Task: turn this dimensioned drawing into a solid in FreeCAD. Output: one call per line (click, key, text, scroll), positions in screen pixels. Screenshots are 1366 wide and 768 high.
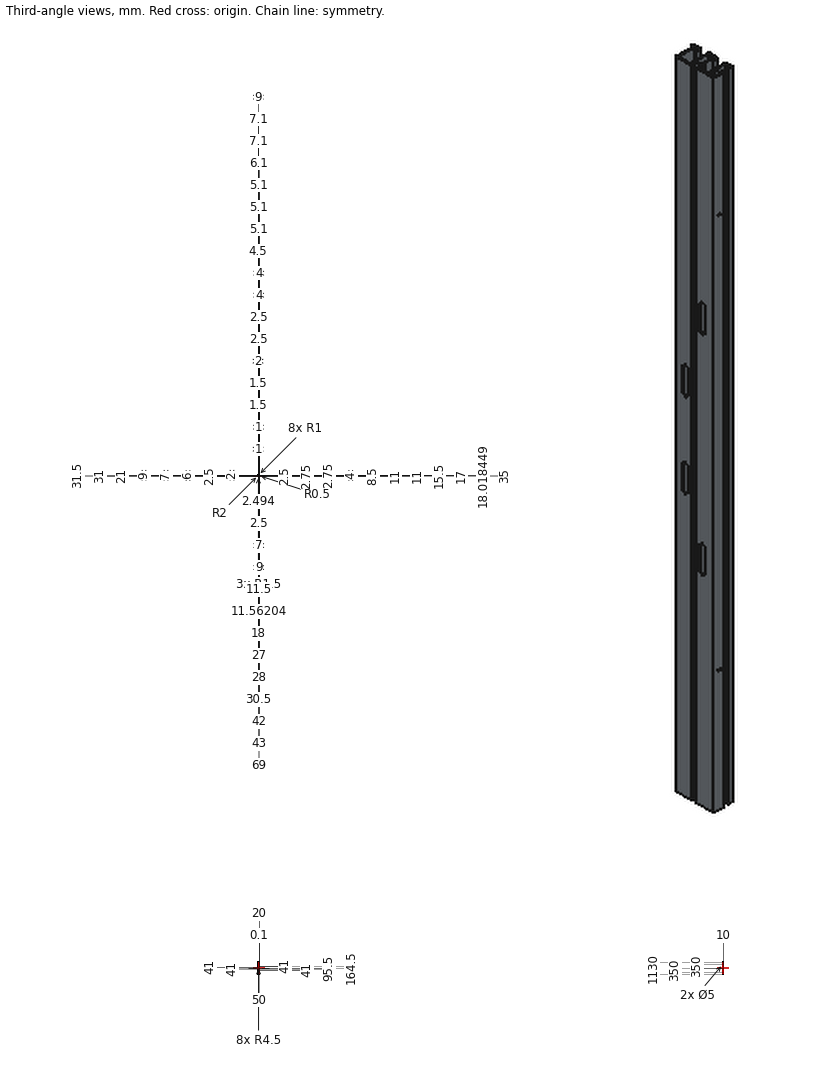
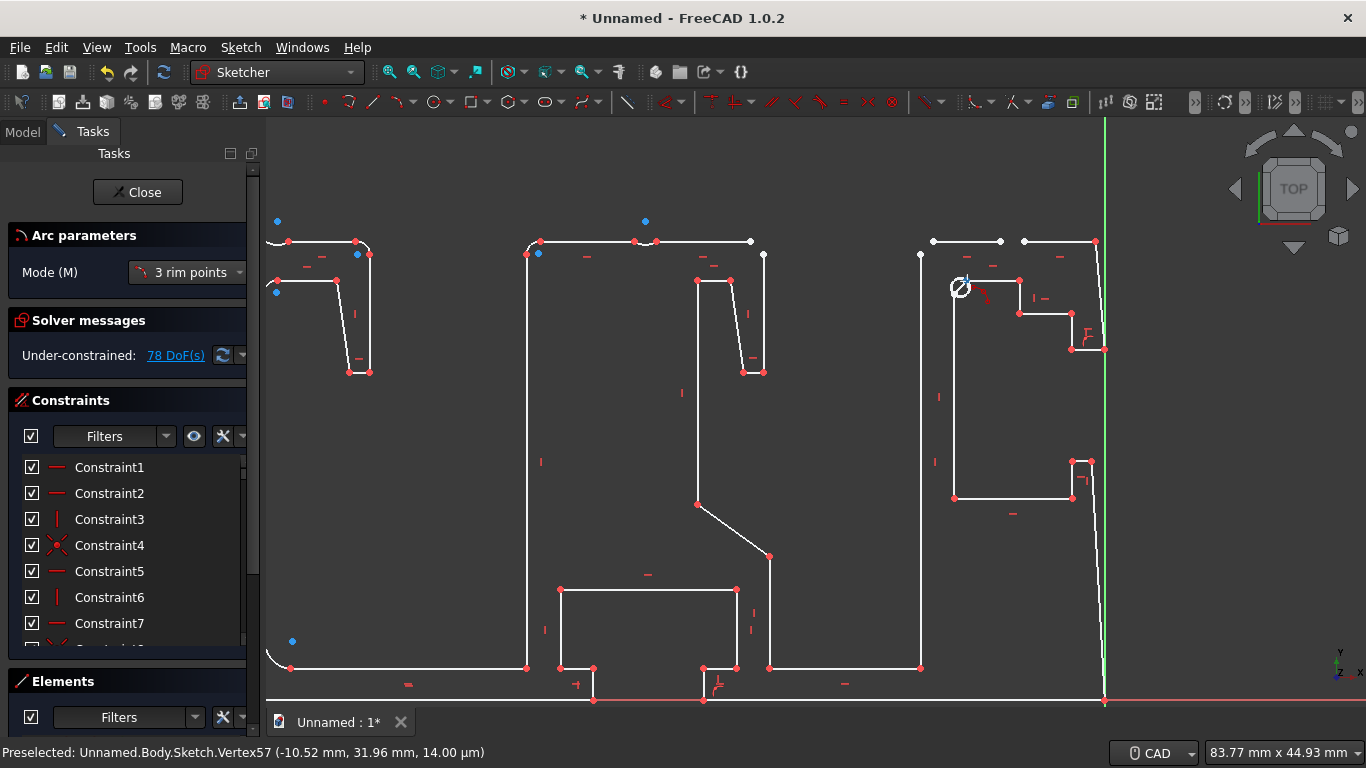
scroll(958, 284, up, 8)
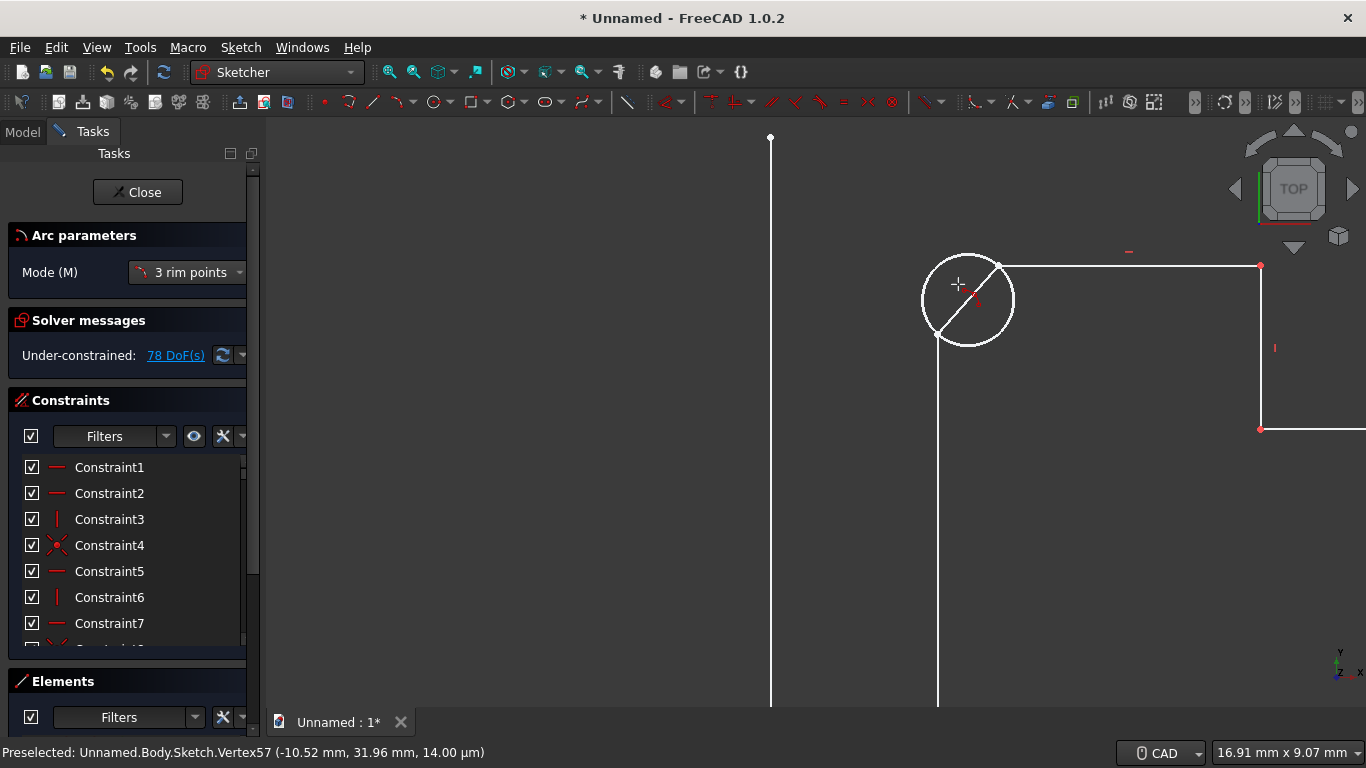
click(954, 282)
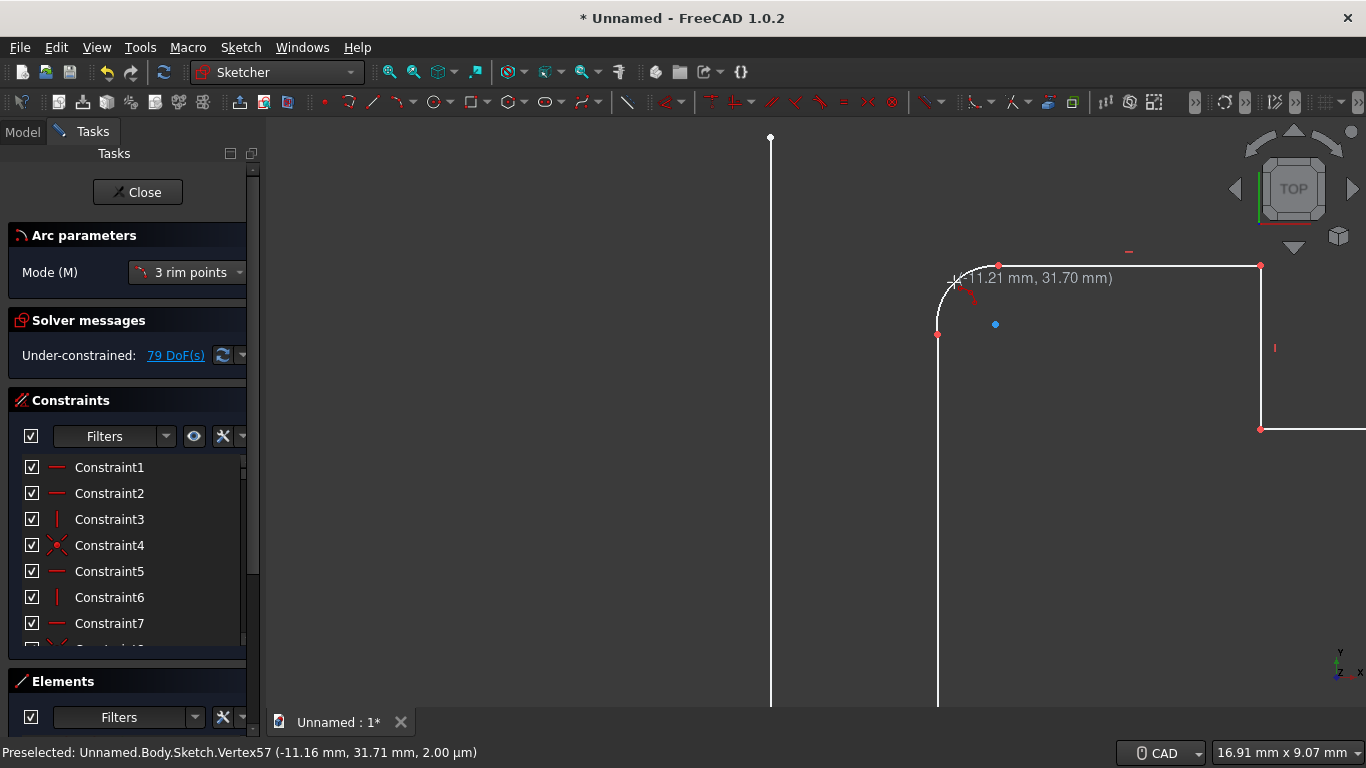
scroll(957, 288, down, 10)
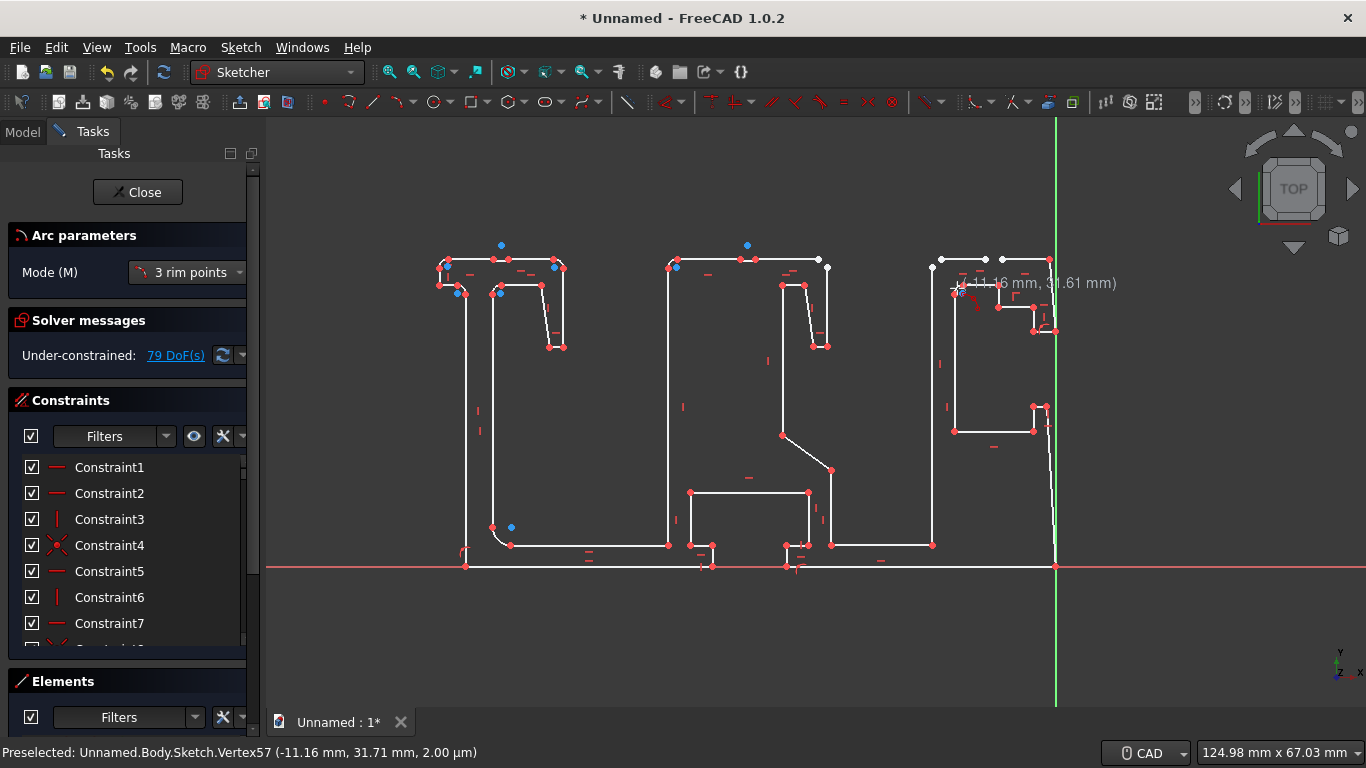
click(1002, 259)
click(986, 259)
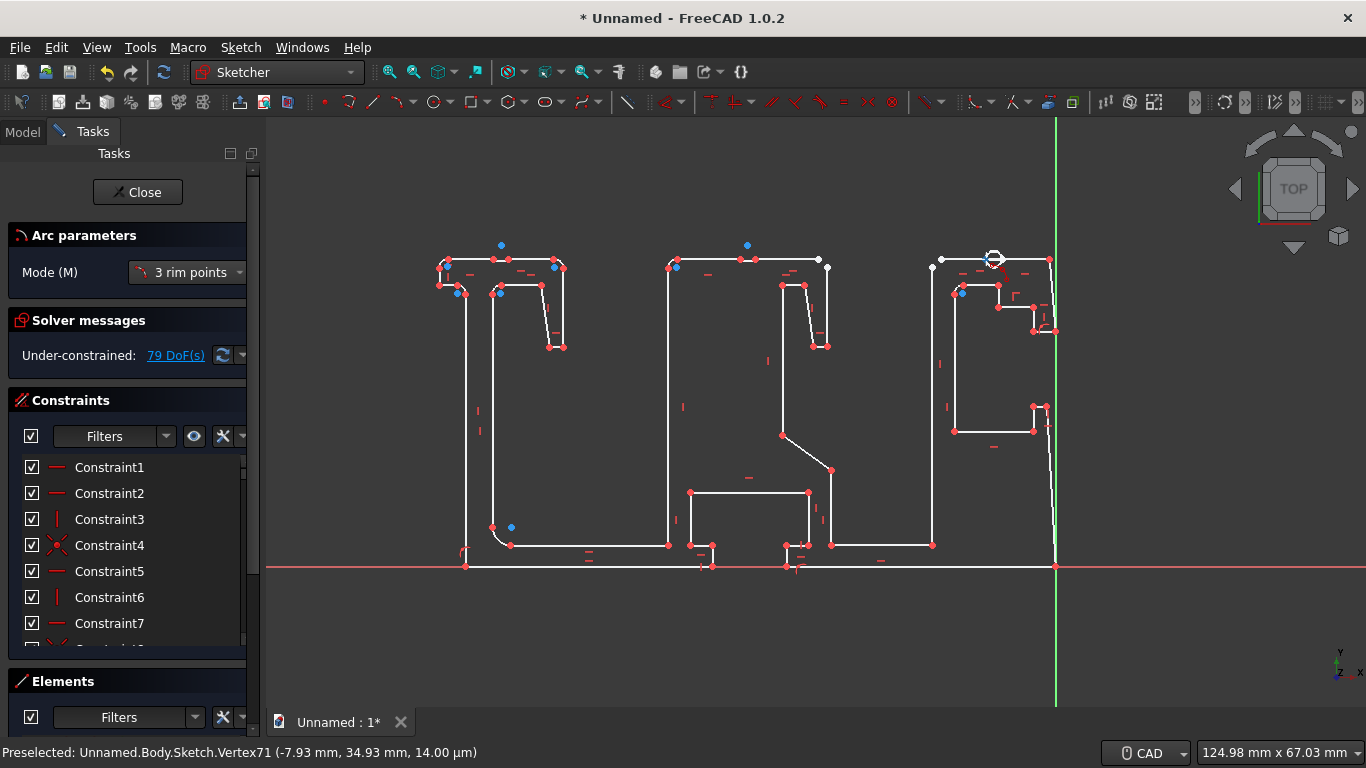
scroll(994, 261, up, 9)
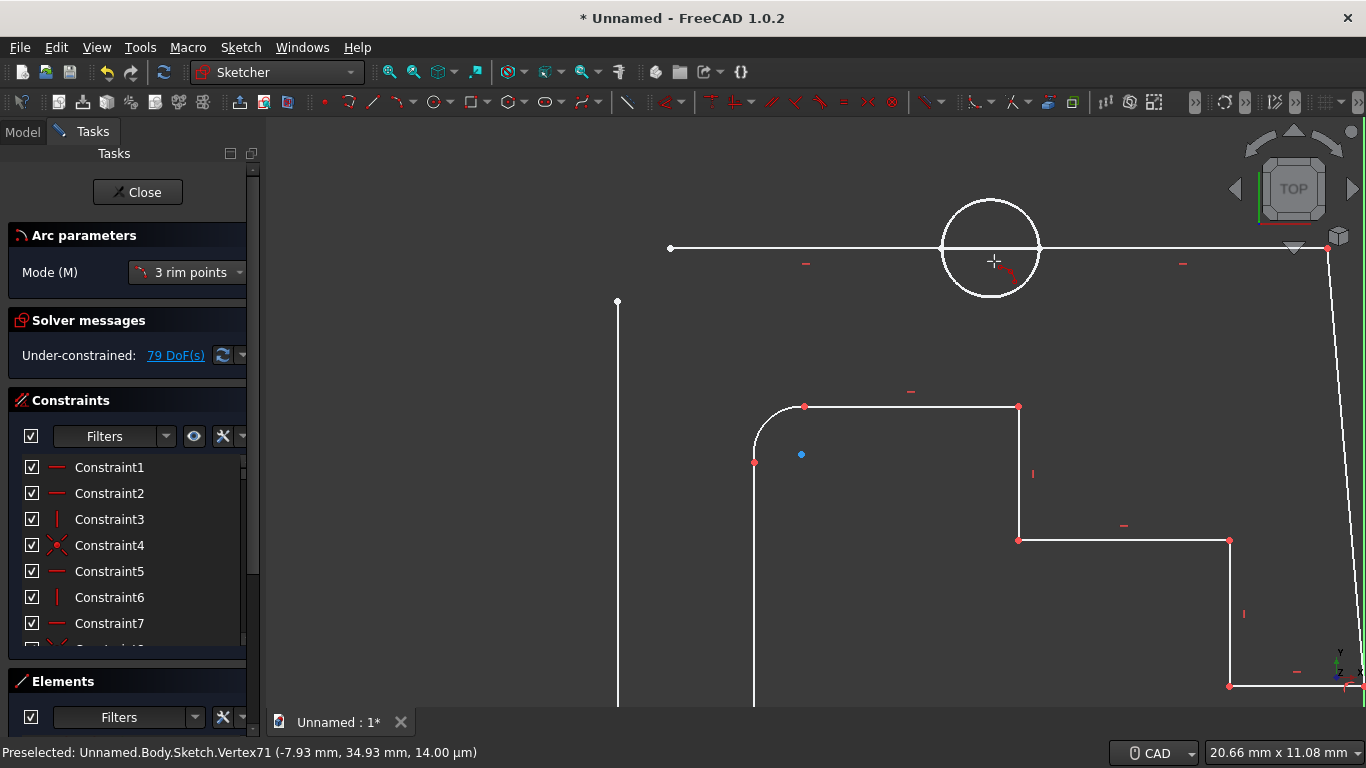
click(992, 261)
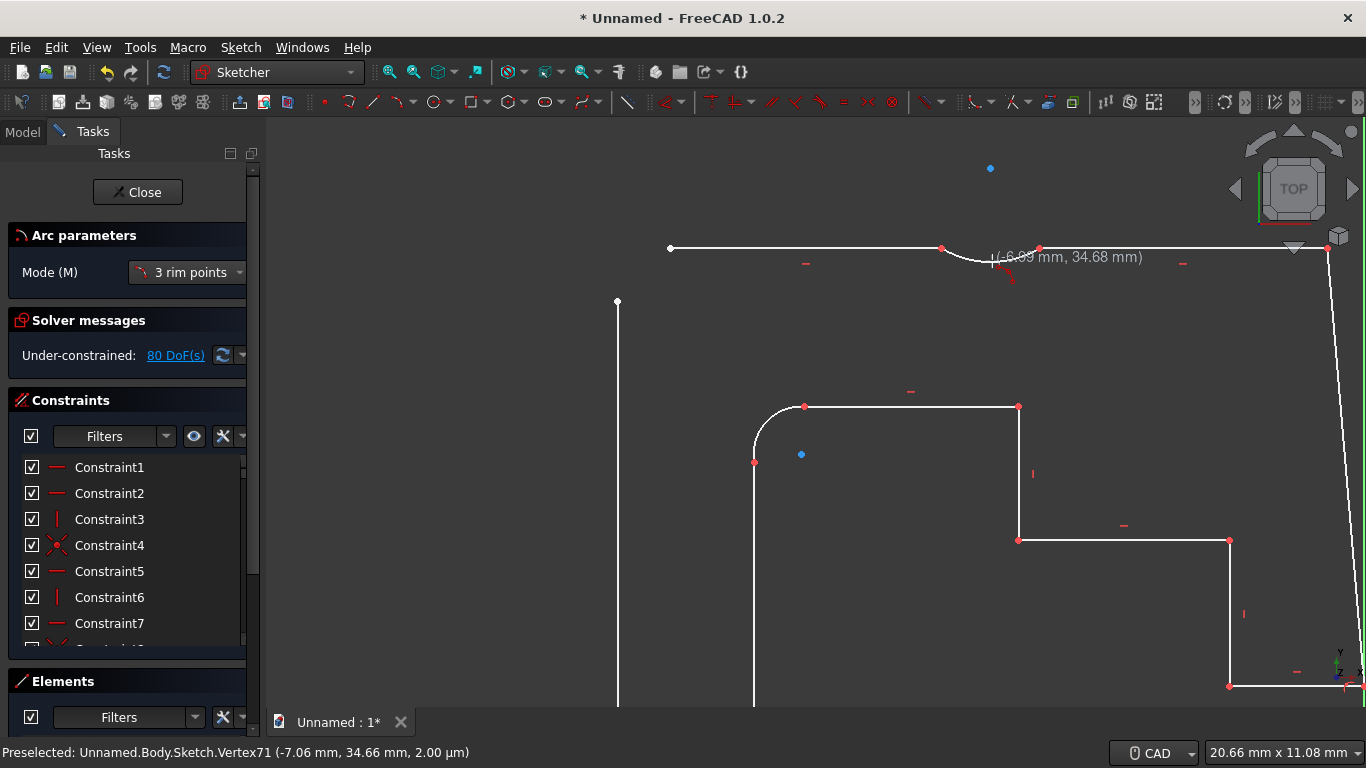
scroll(994, 261, down, 9)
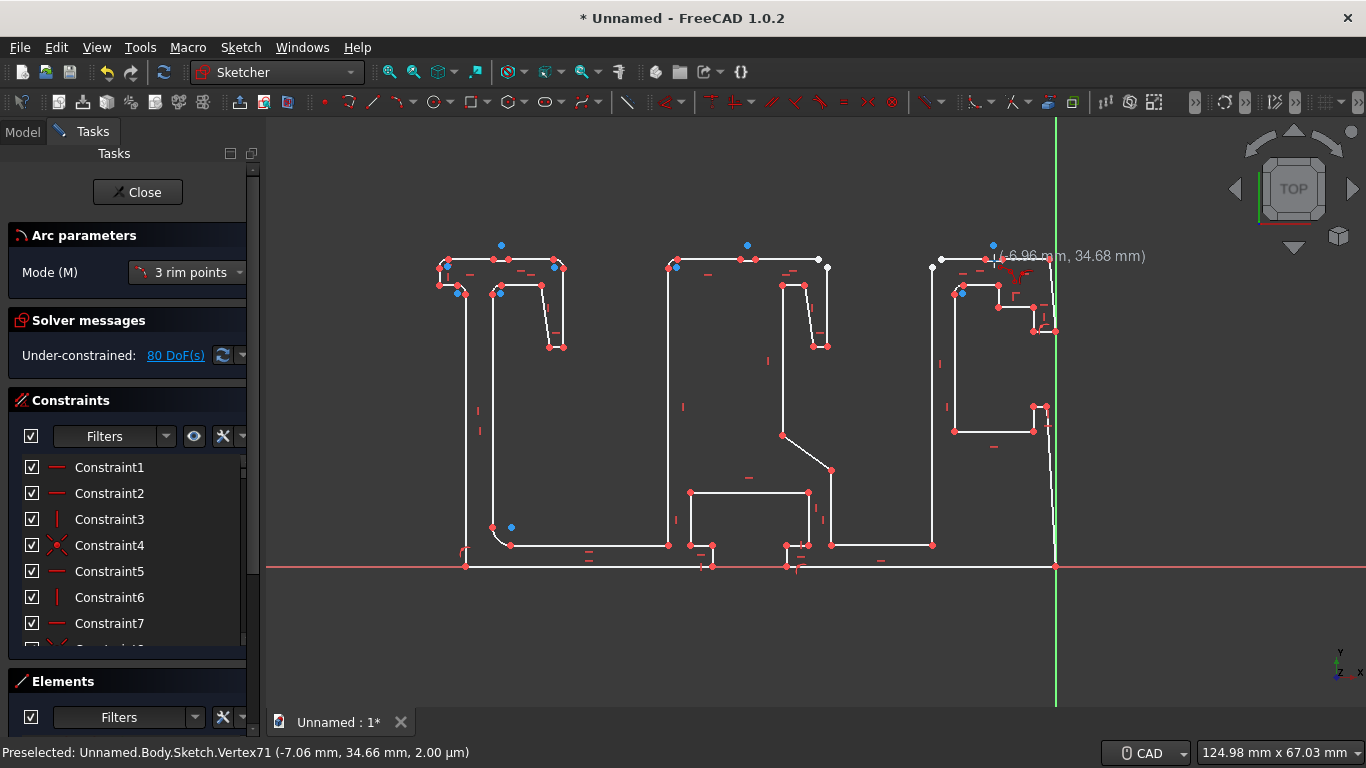
scroll(941, 259, up, 2)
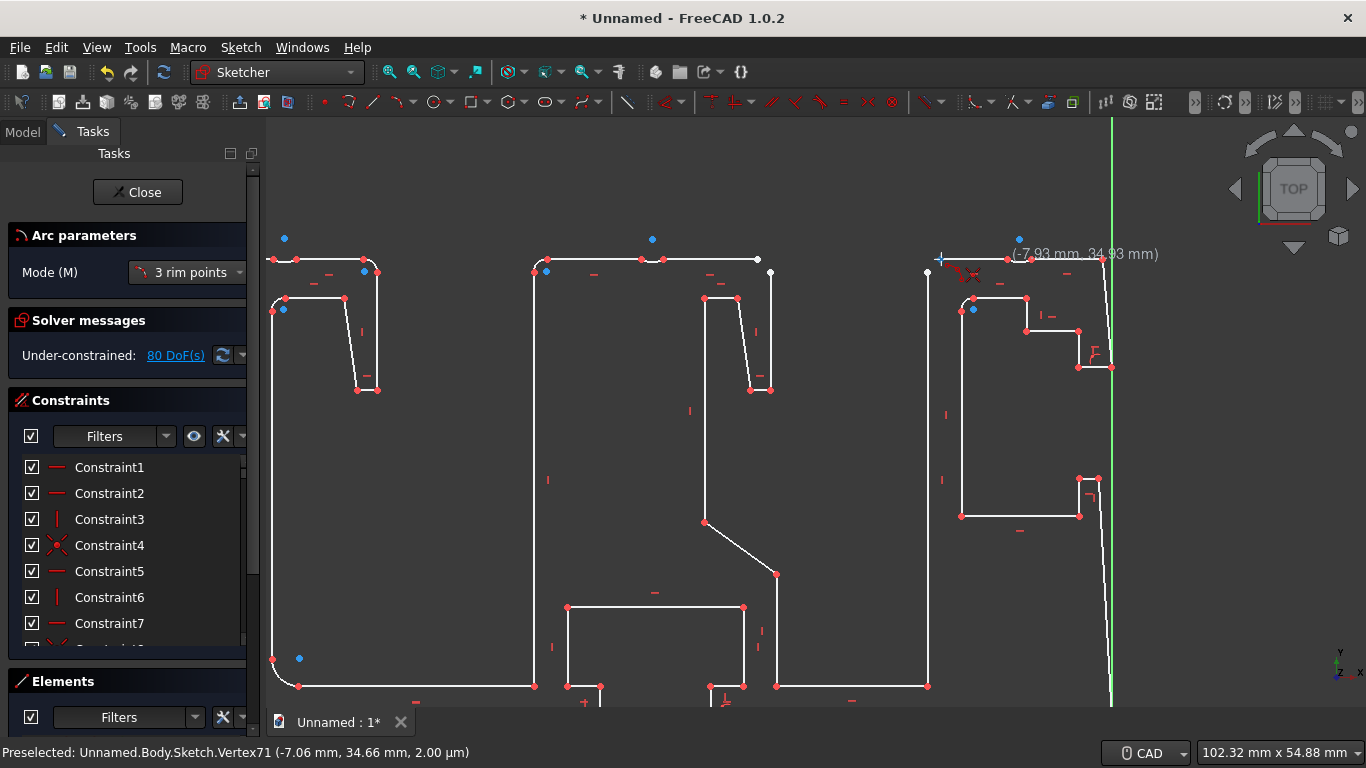
click(941, 259)
click(928, 272)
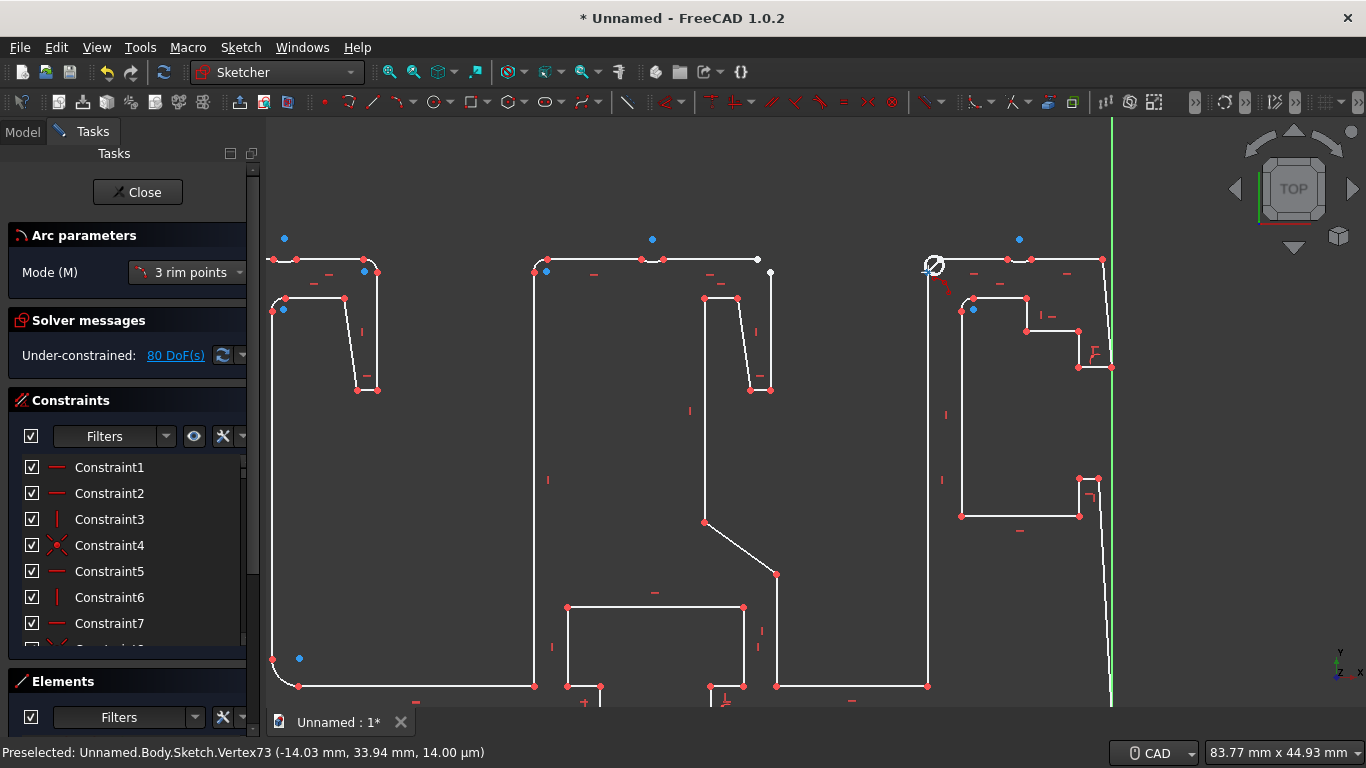
scroll(932, 262, up, 8)